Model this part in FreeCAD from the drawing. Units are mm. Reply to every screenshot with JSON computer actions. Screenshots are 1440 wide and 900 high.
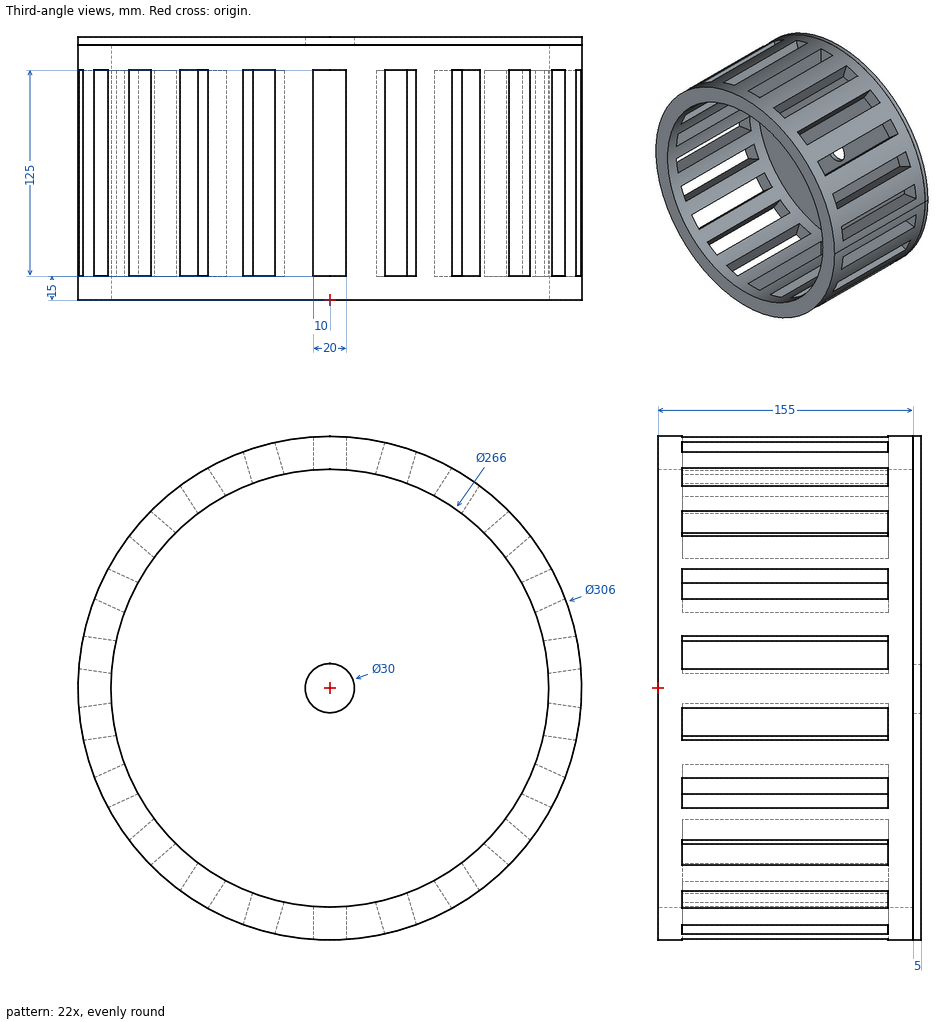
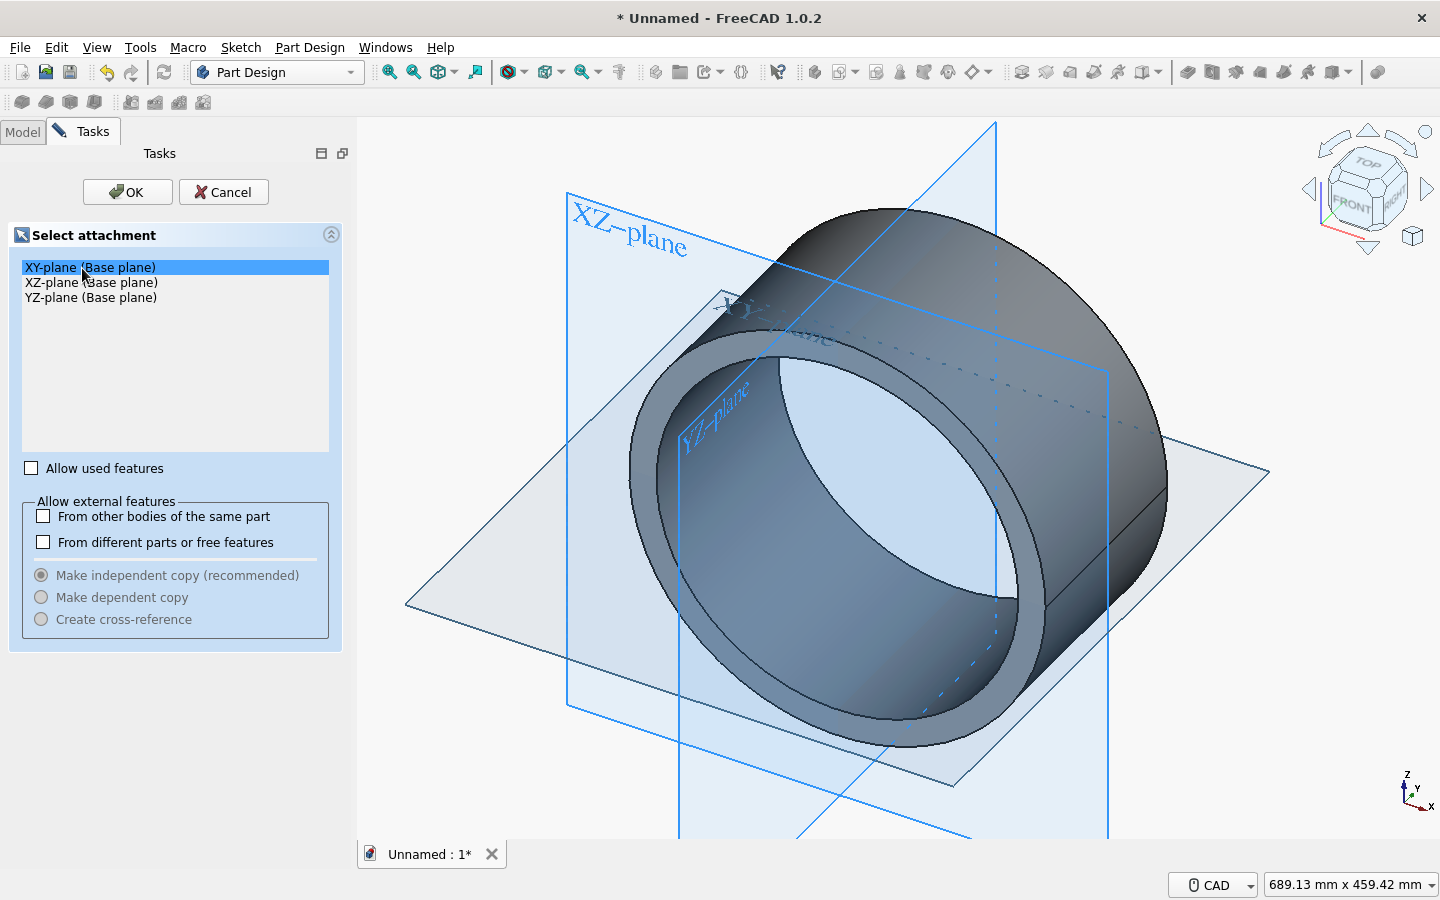
{"action": "left_click", "coordinate": [128, 192]}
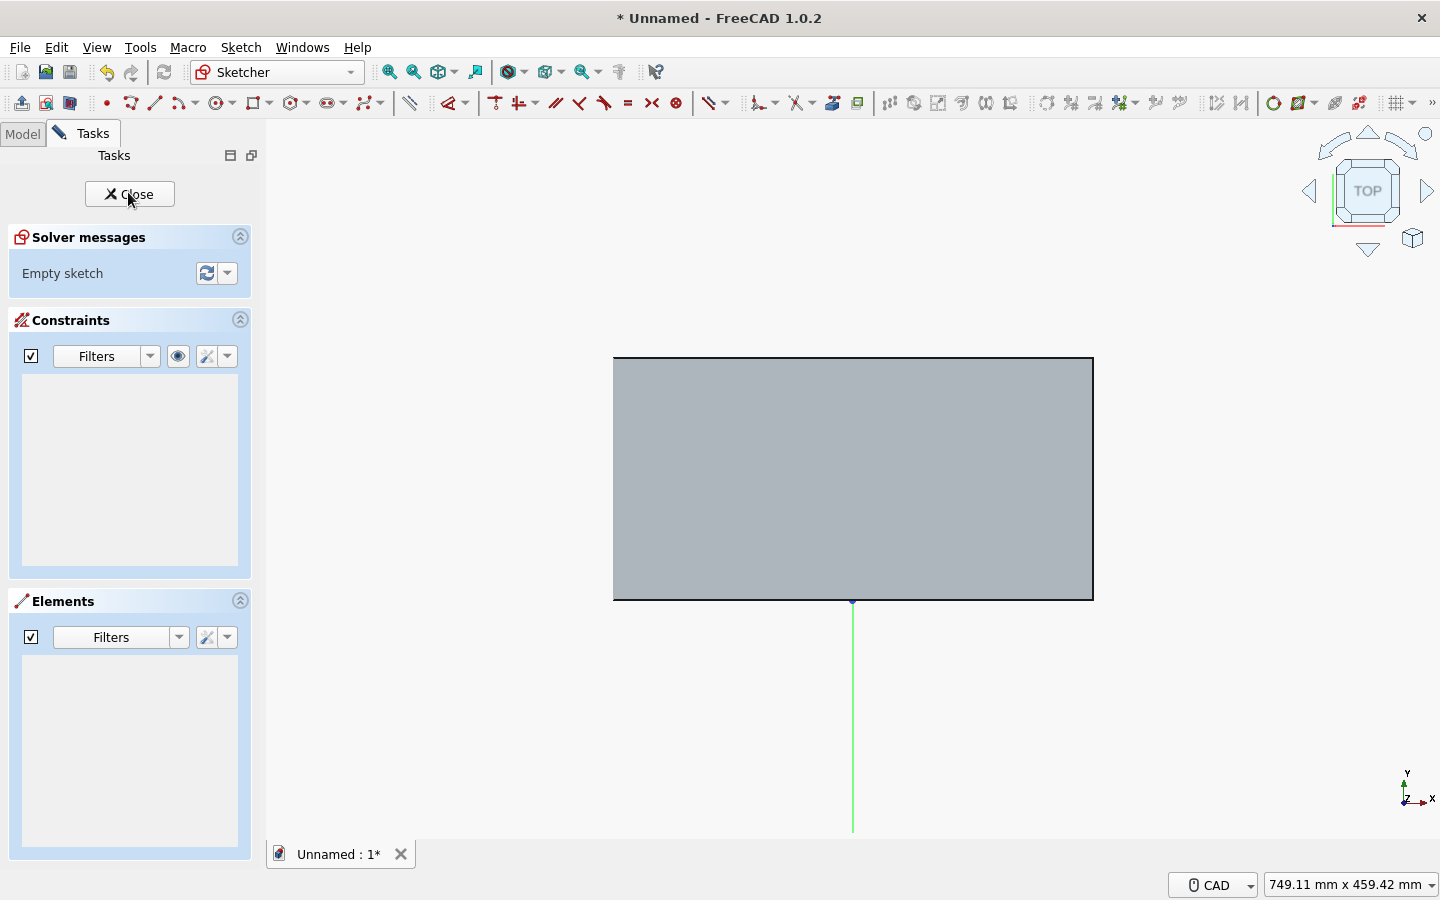
{"action": "left_click", "coordinate": [70, 104]}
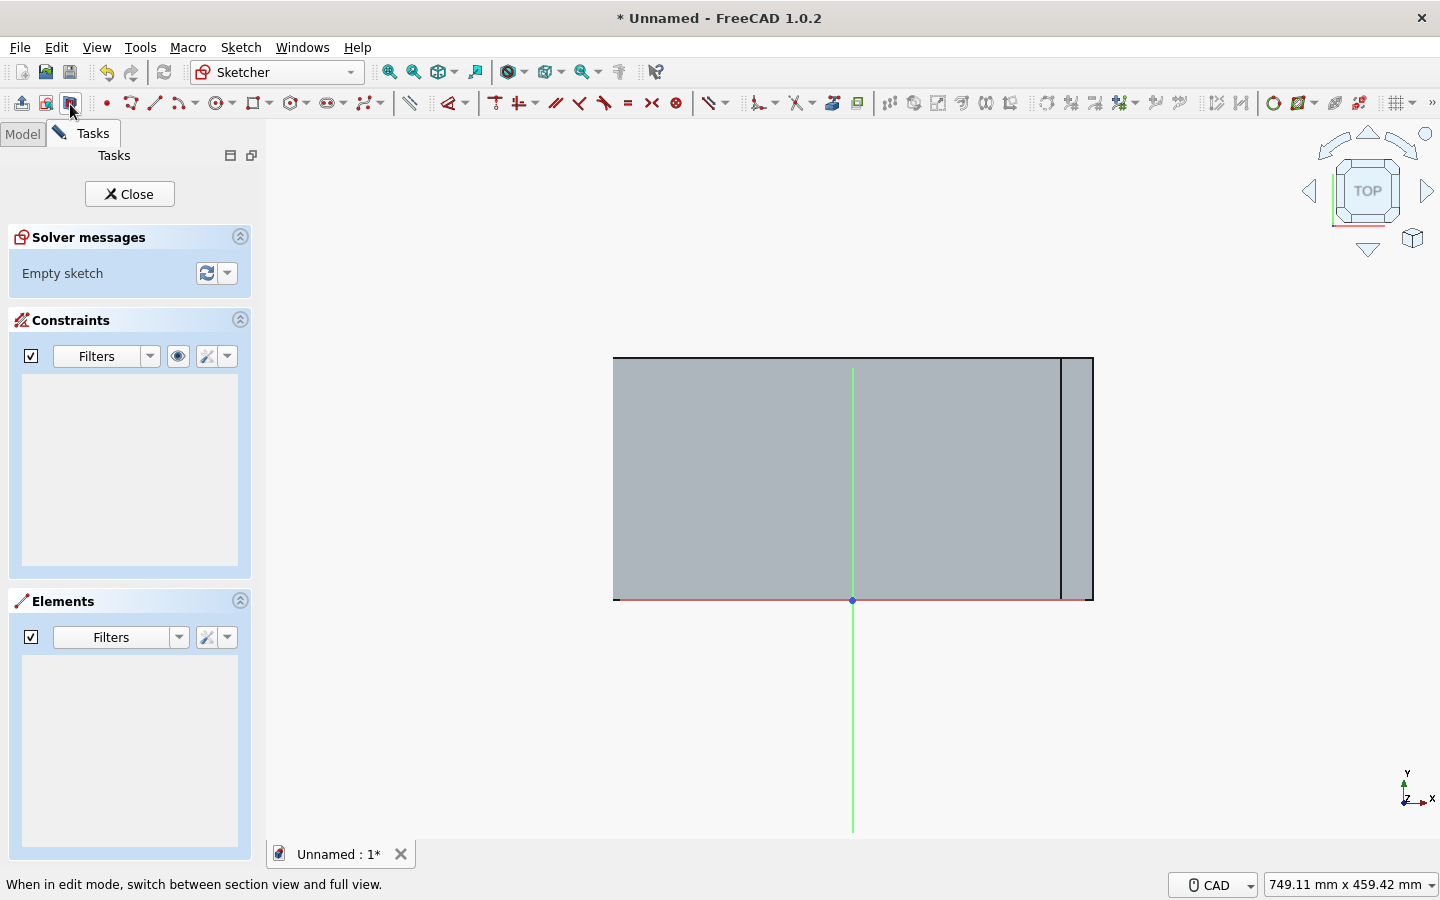
{"action": "scroll", "coordinate": [909, 500], "scroll_direction": "up", "scroll_amount": 4}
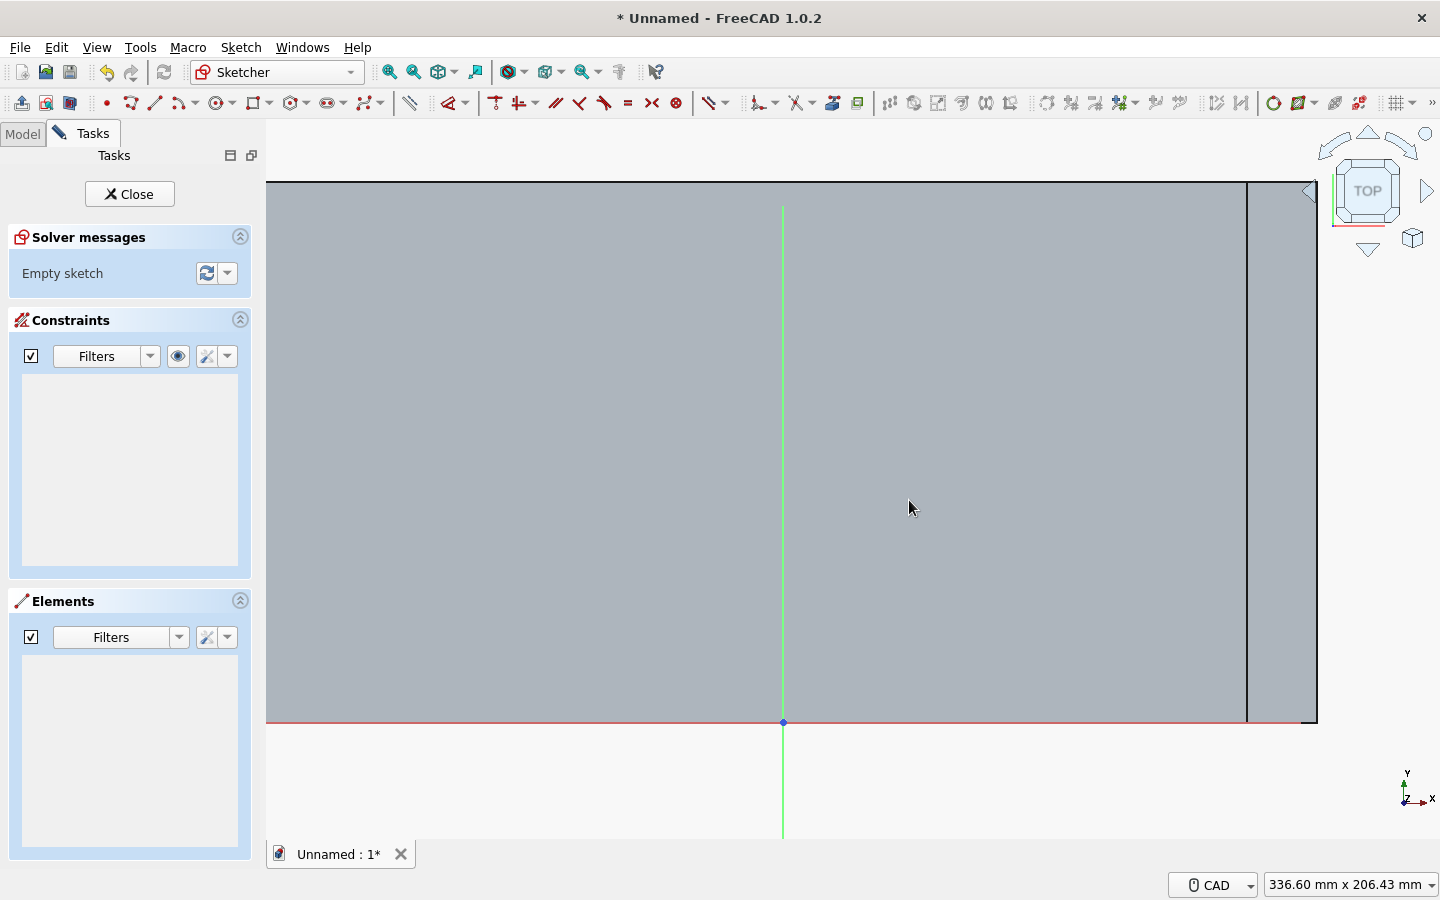
{"action": "left_click", "coordinate": [254, 104]}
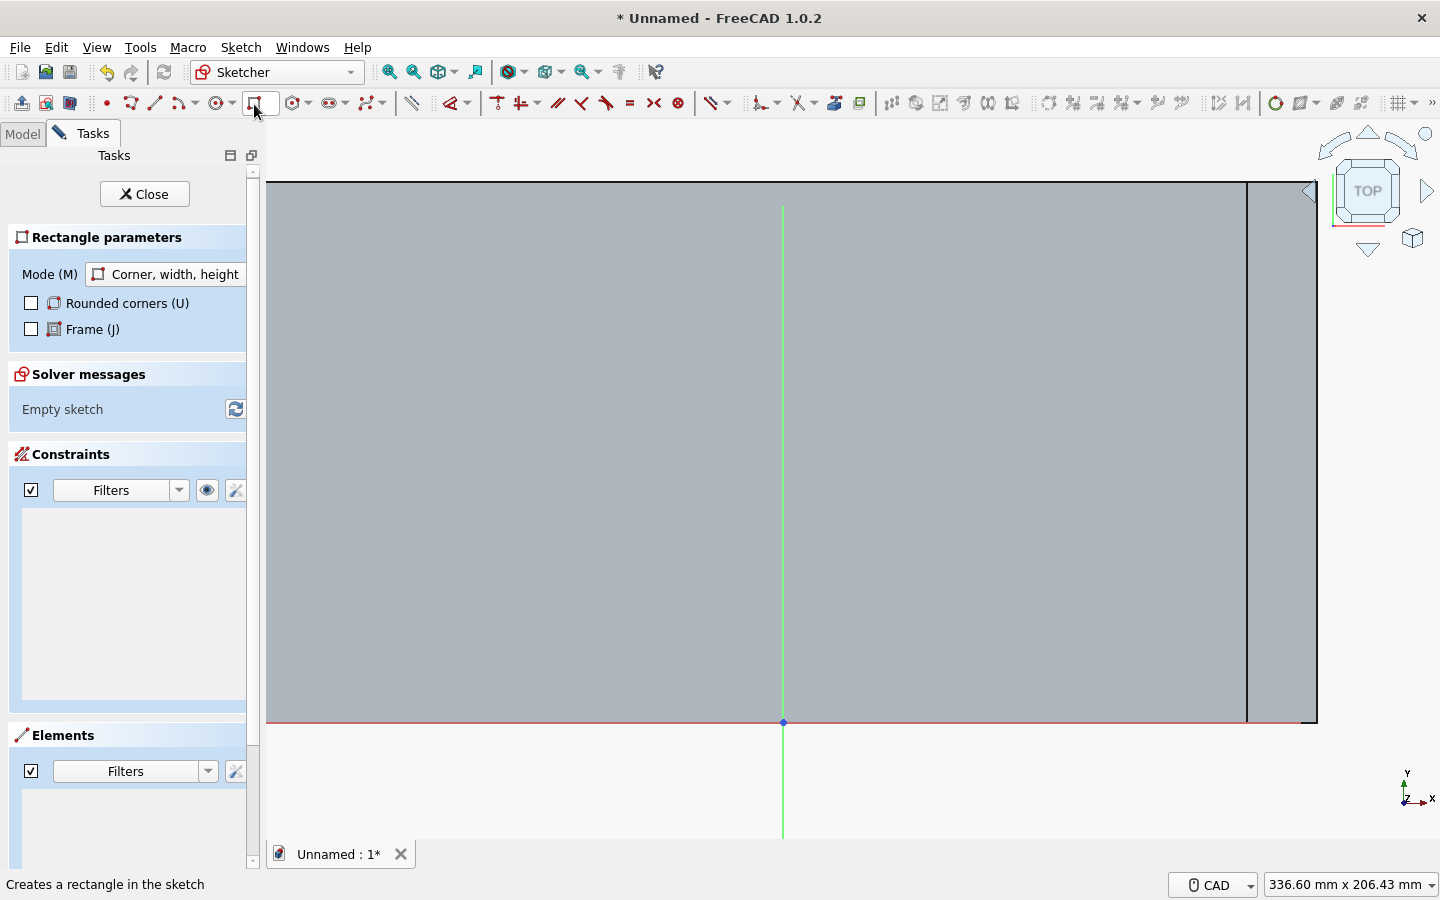
{"action": "left_click", "coordinate": [748, 235]}
{"action": "left_click", "coordinate": [818, 671]}
{"action": "key", "text": "Escape"}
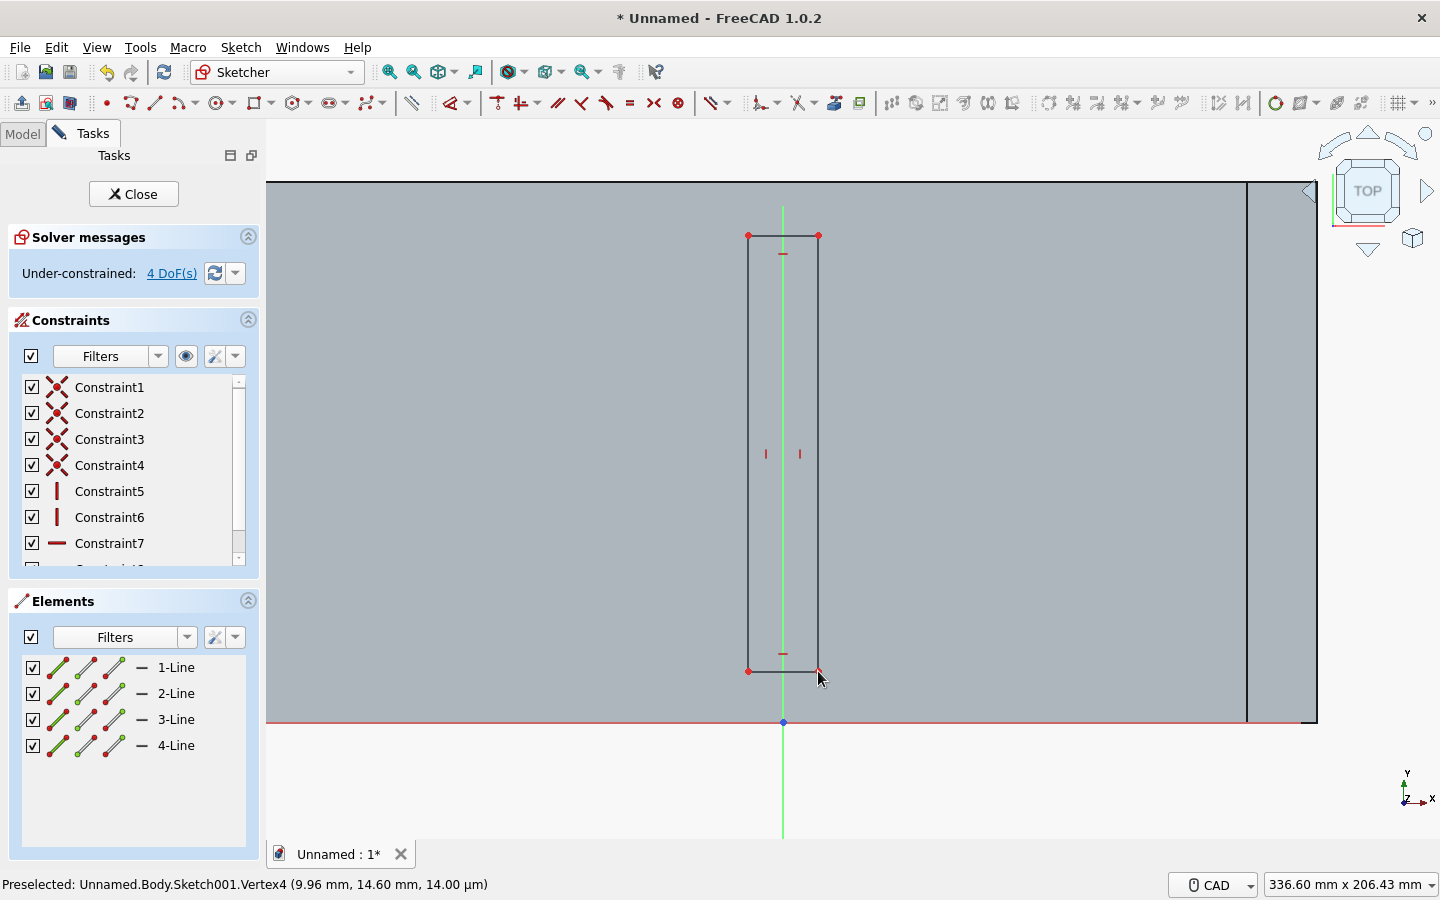
{"action": "left_click", "coordinate": [450, 104]}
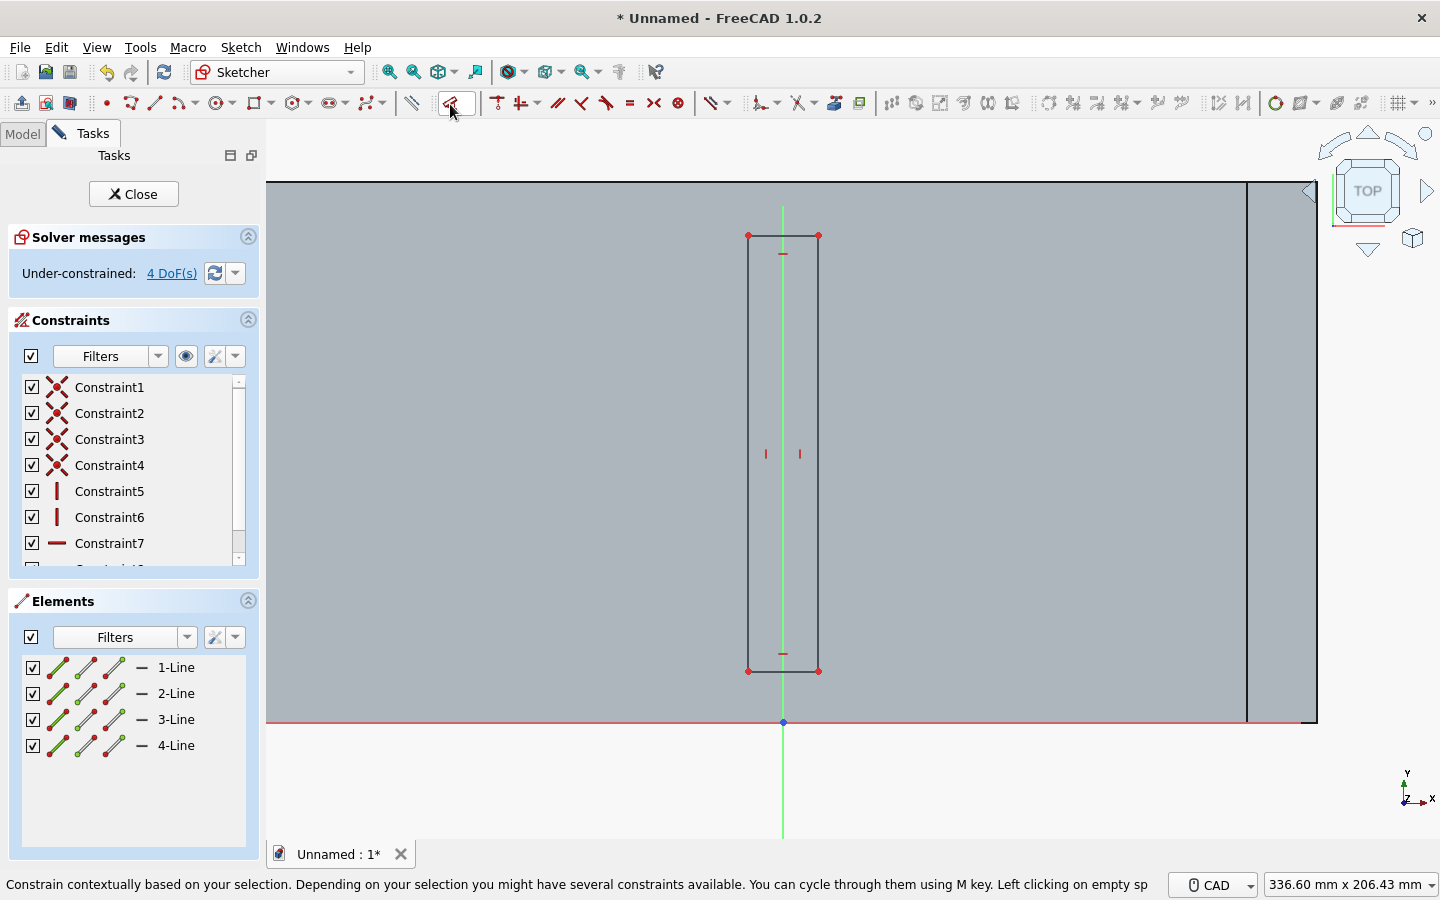
{"action": "left_click", "coordinate": [769, 672]}
{"action": "left_click", "coordinate": [767, 706]}